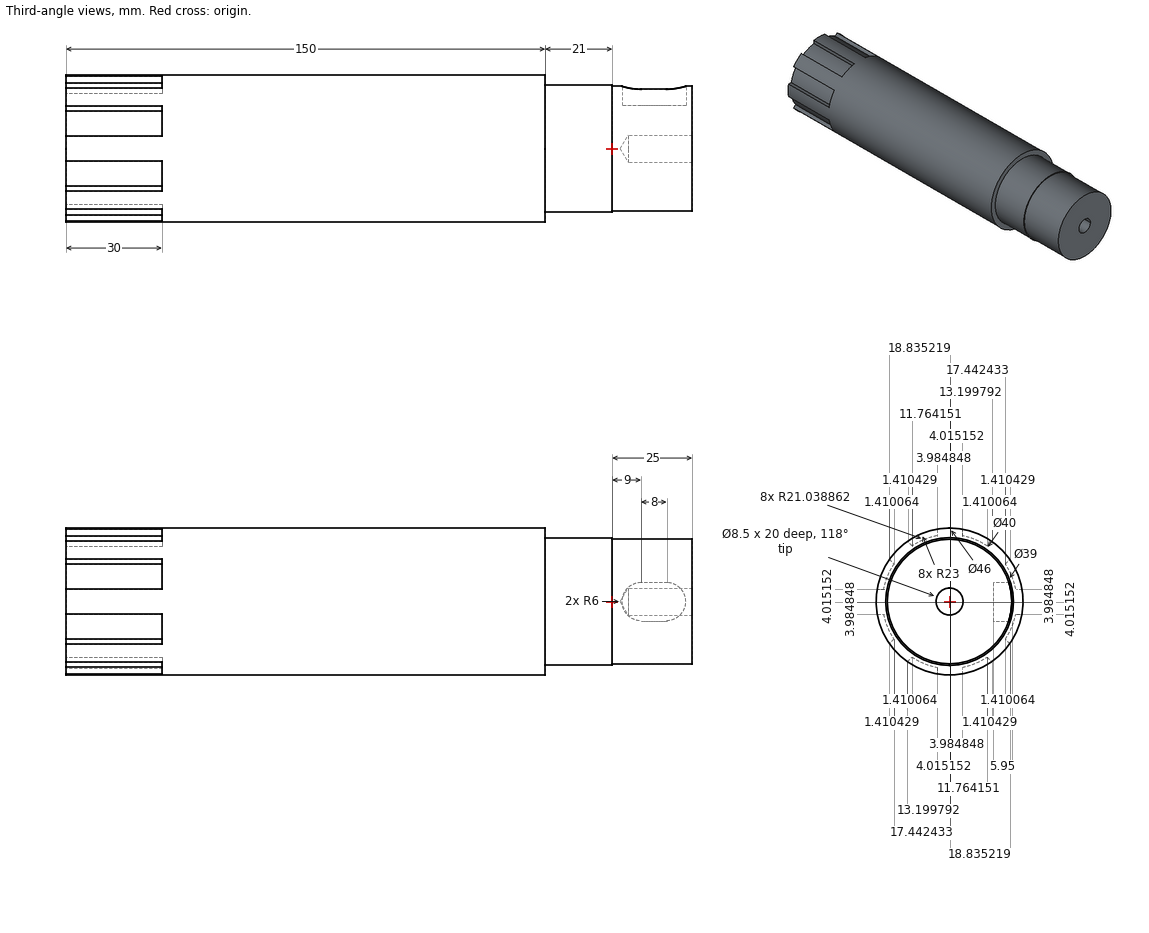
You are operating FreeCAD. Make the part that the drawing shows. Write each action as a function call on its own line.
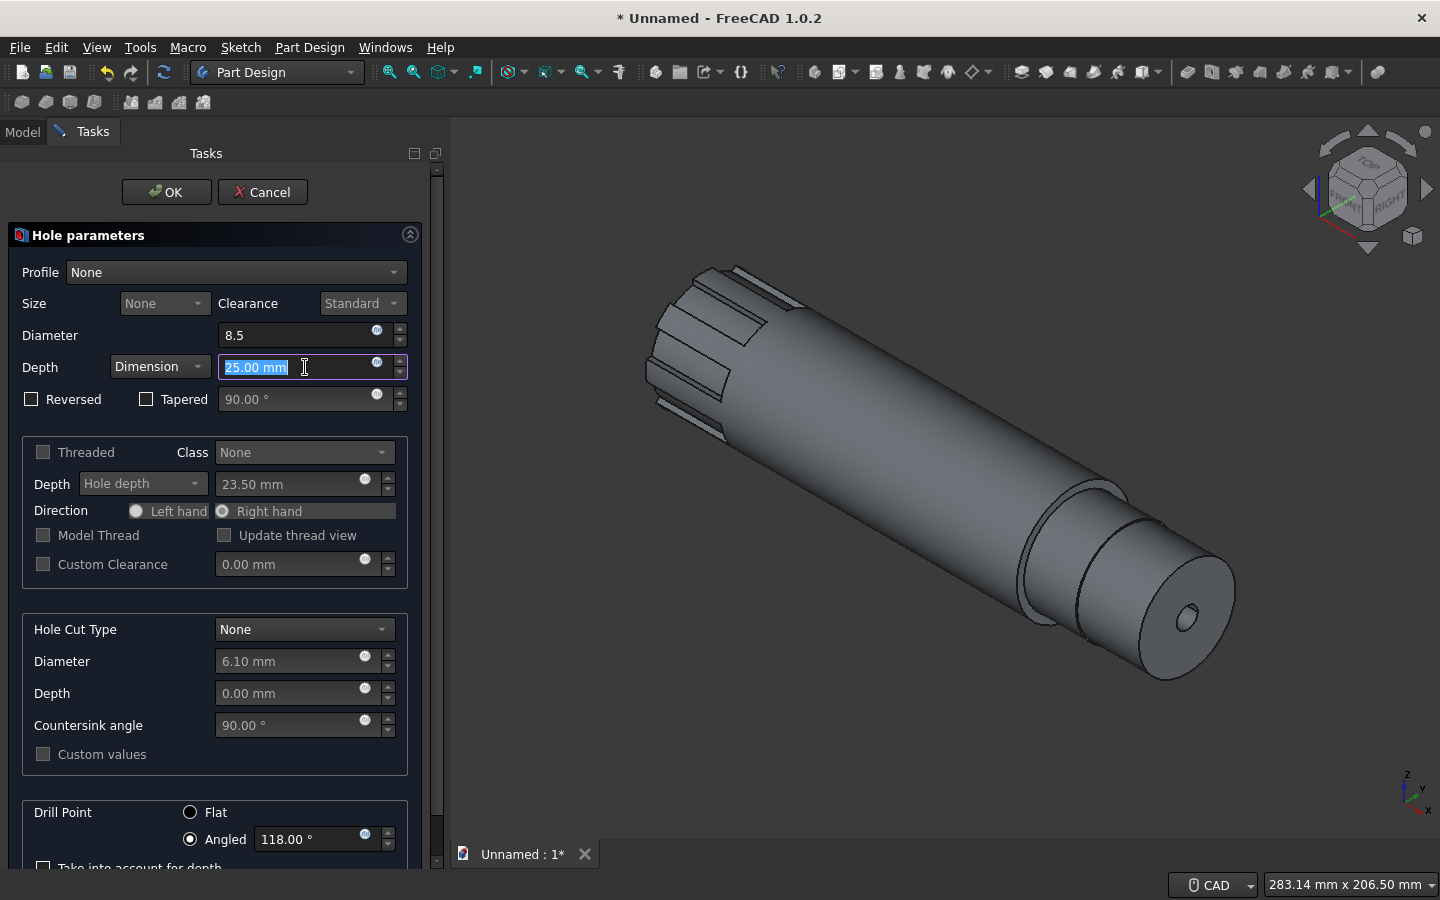
text(20)
key(Tab)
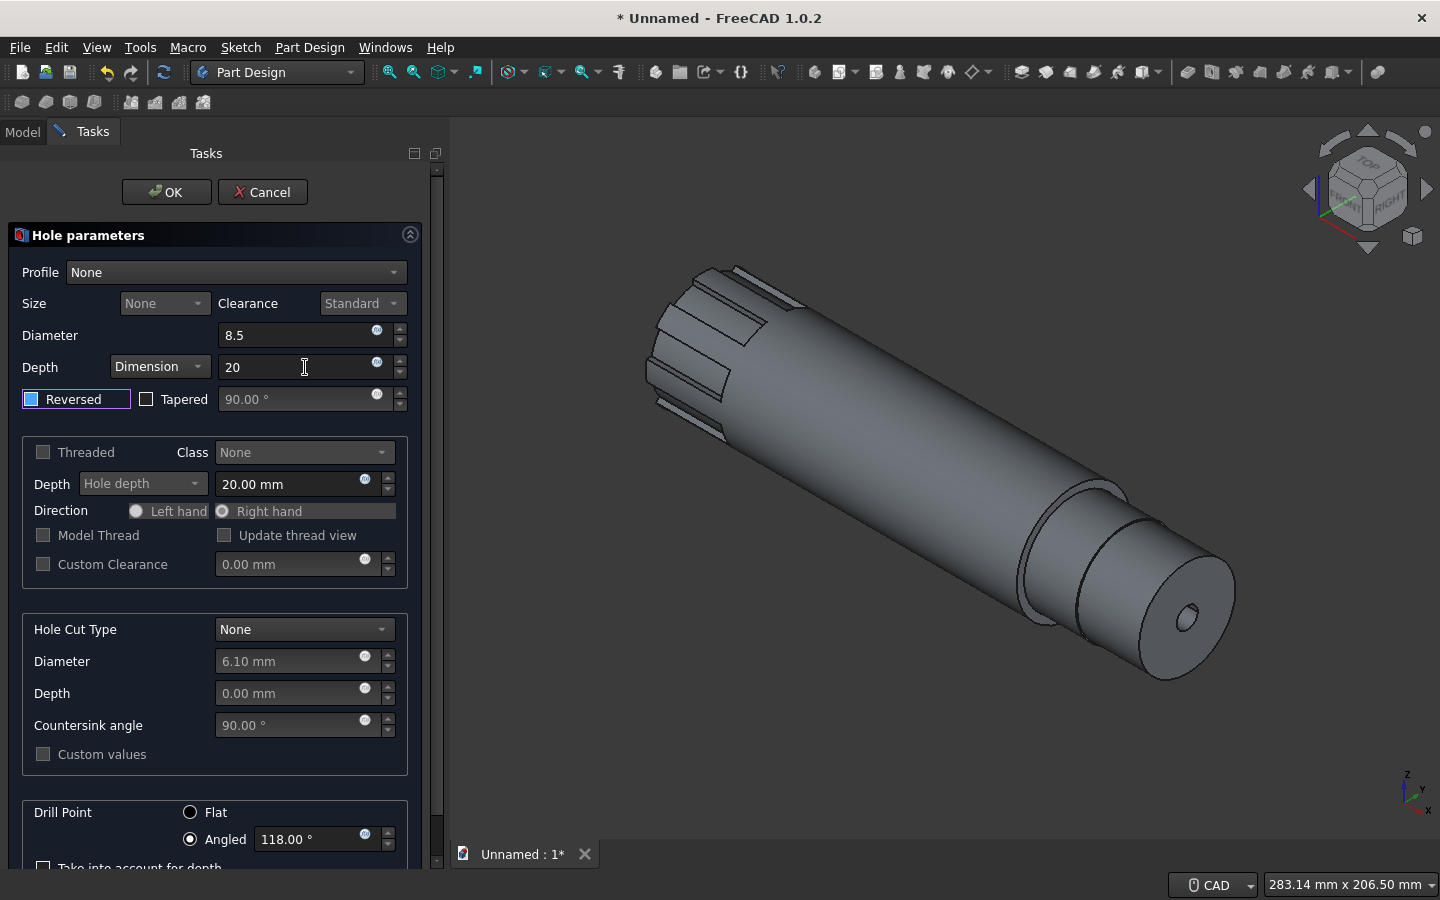
click(167, 192)